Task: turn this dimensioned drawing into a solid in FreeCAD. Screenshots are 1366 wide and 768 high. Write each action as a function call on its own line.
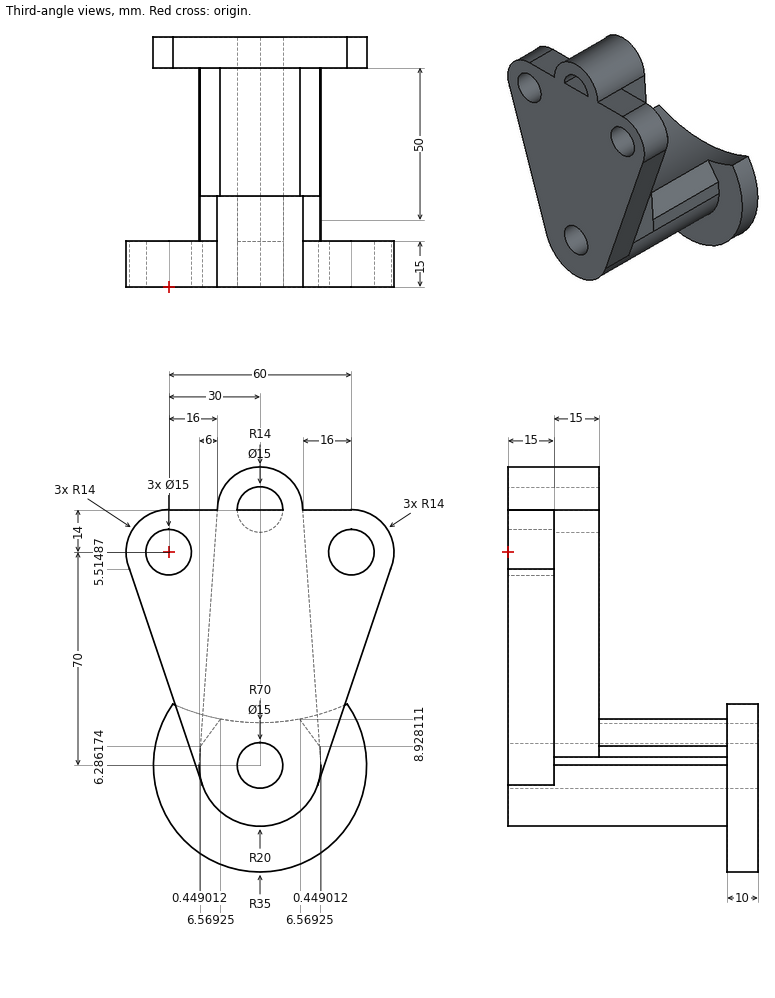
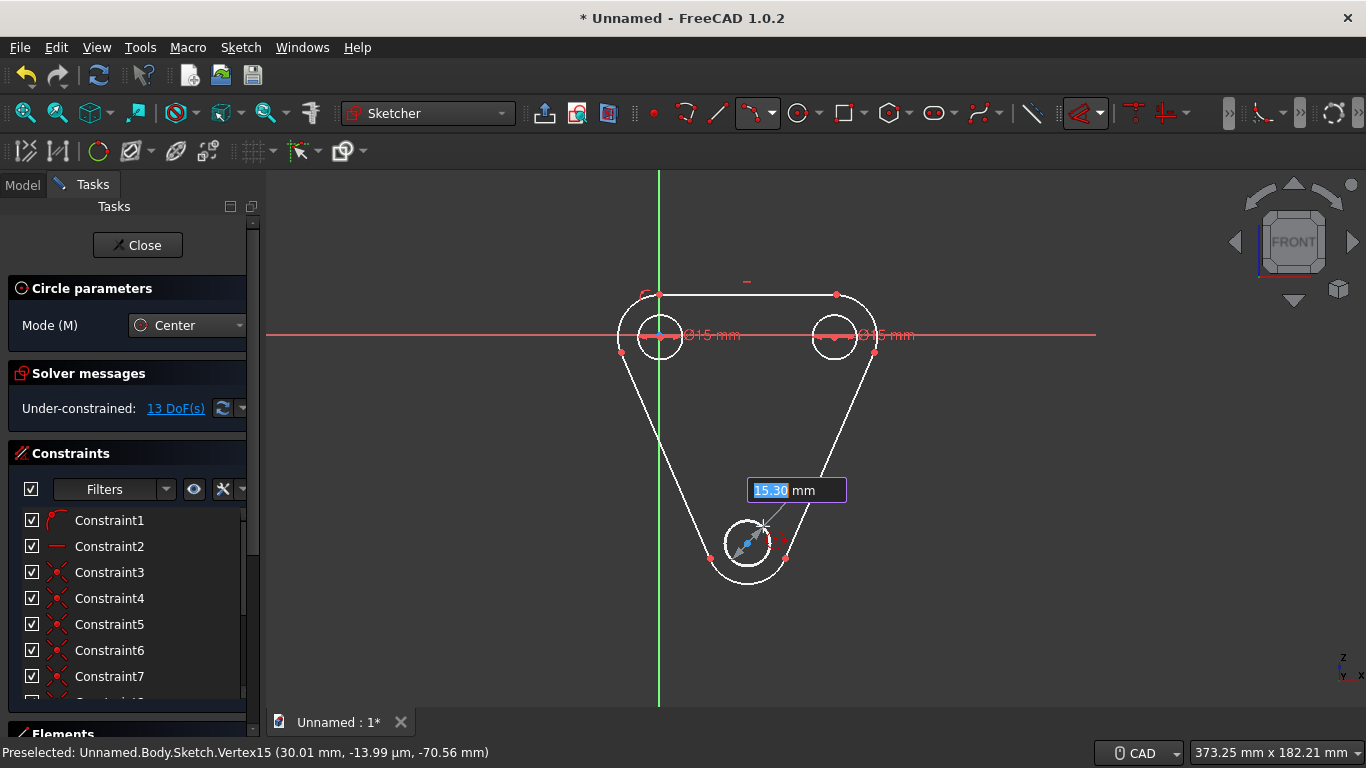
text(15)
key(Return)
key(Escape)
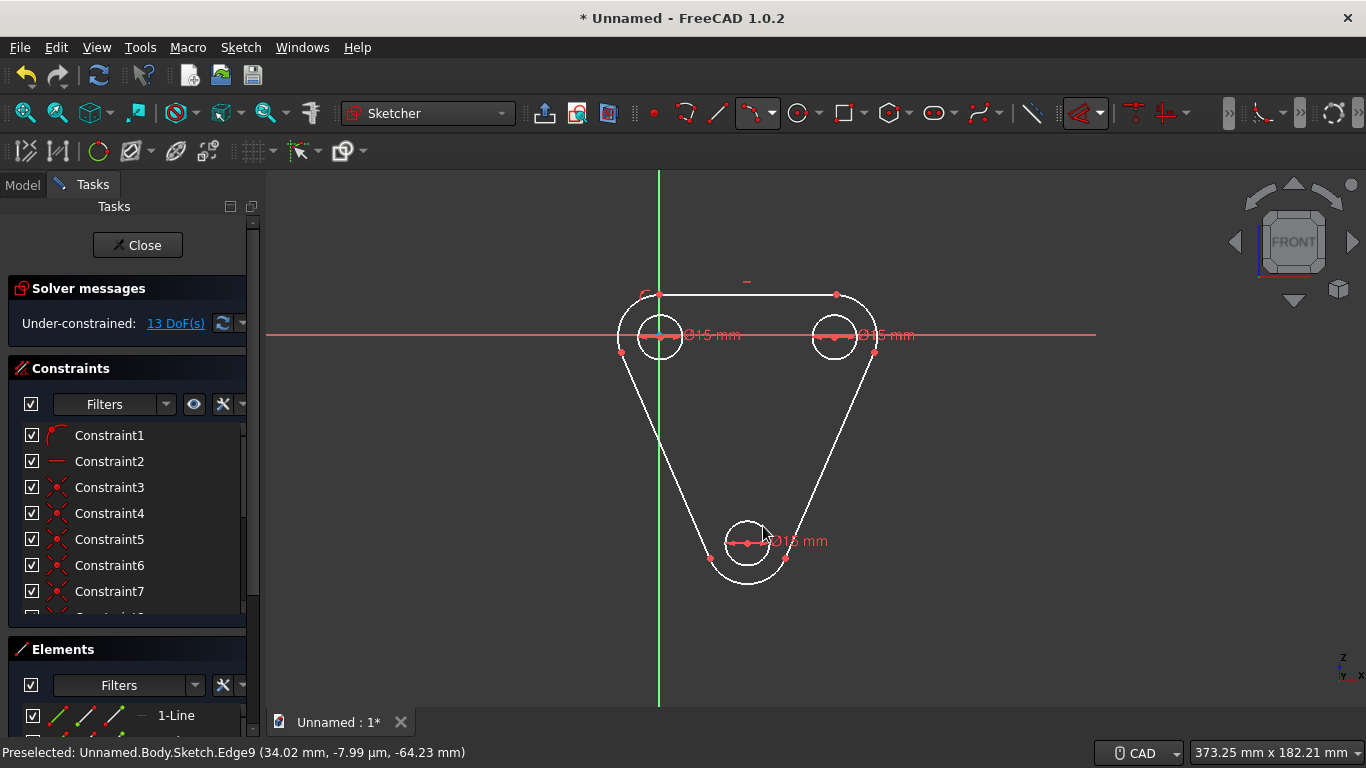
click(683, 497)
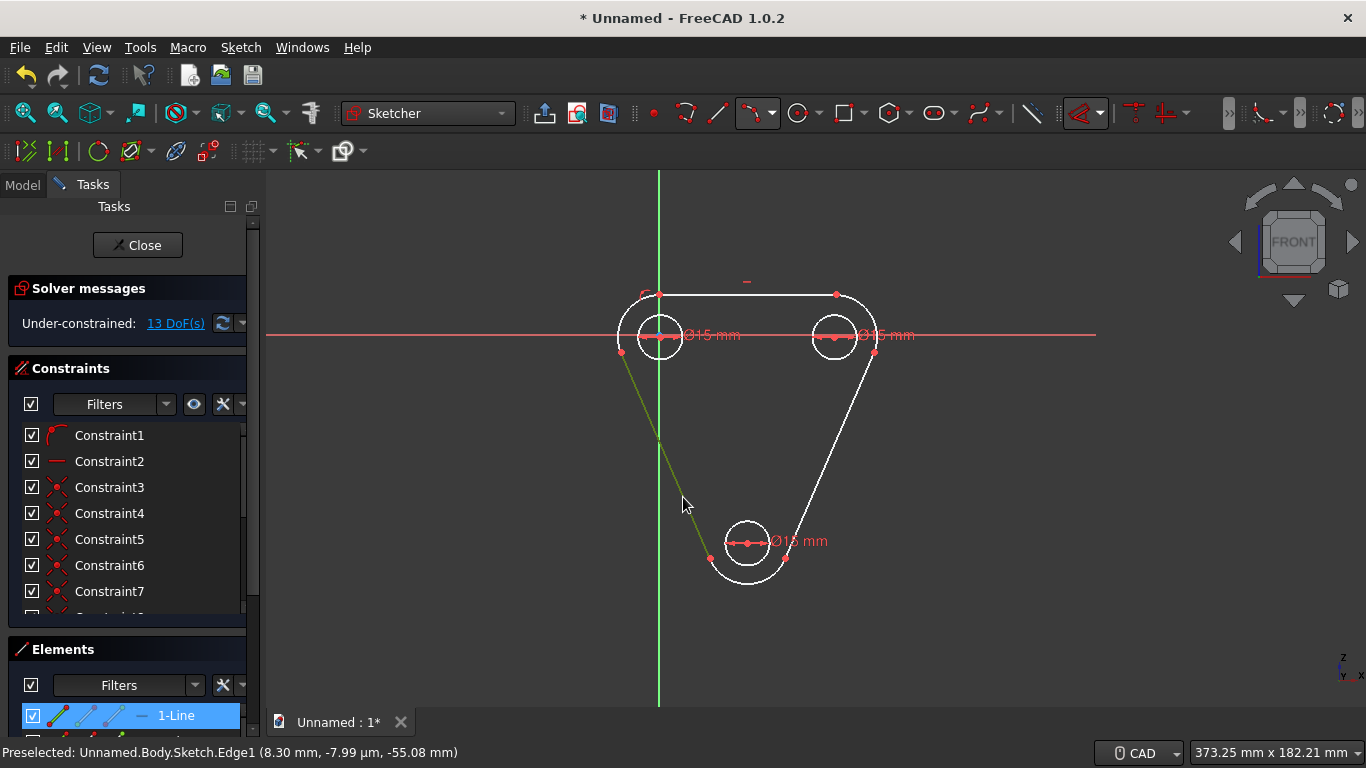
click(636, 303)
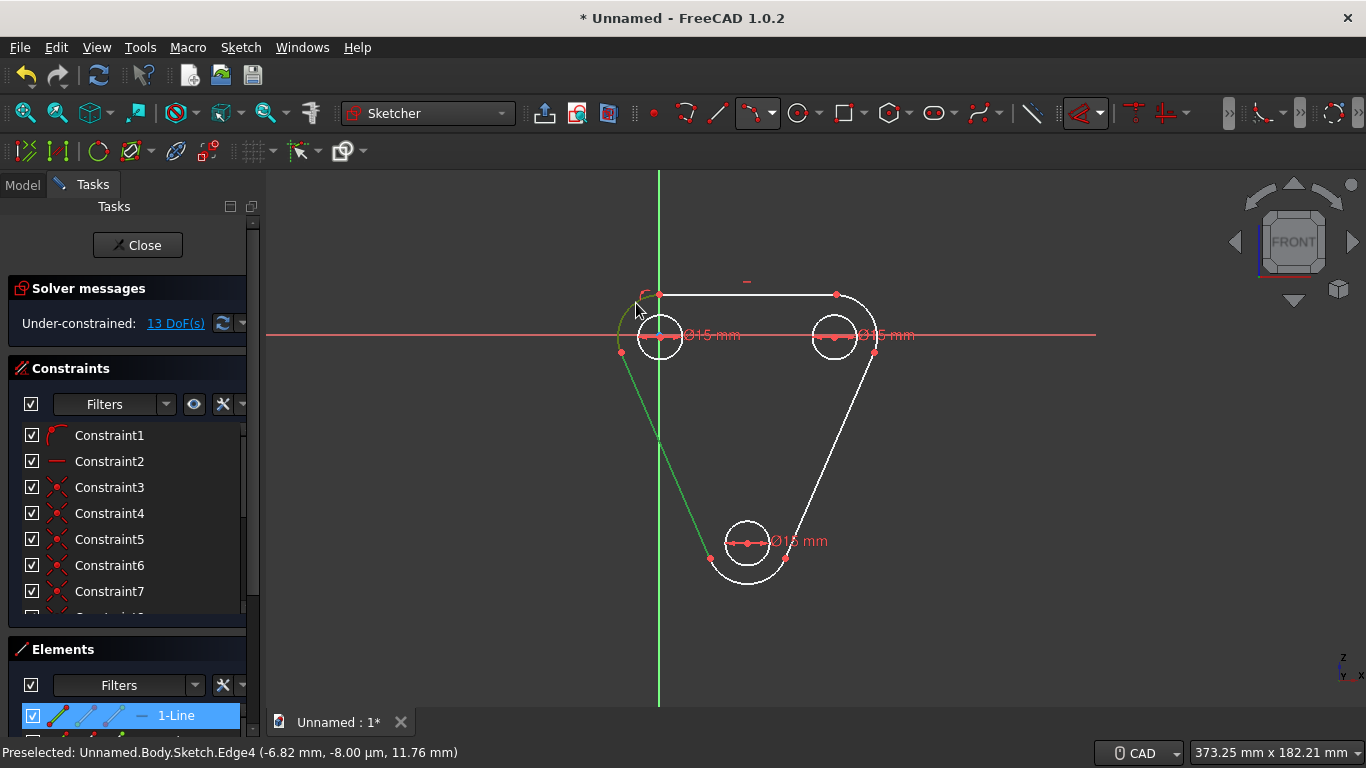
key(t)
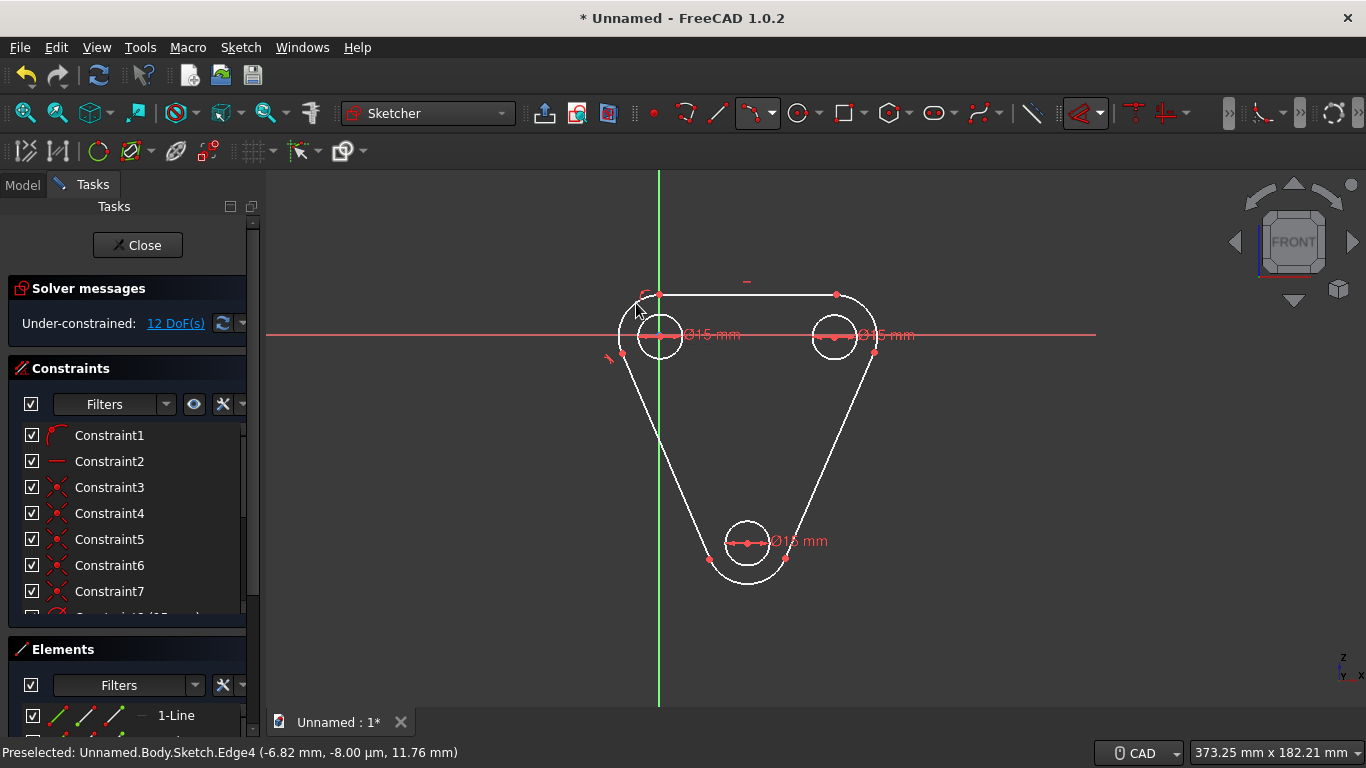
click(684, 497)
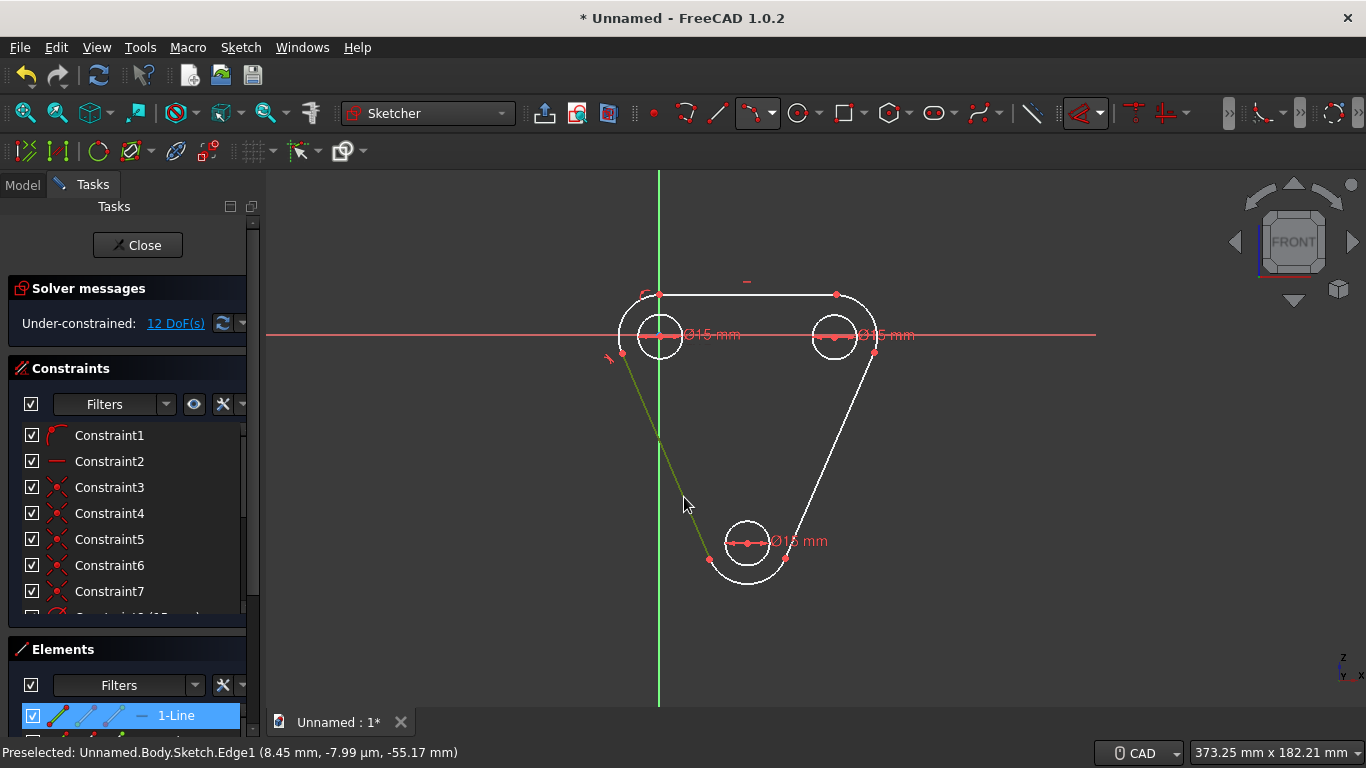
click(729, 580)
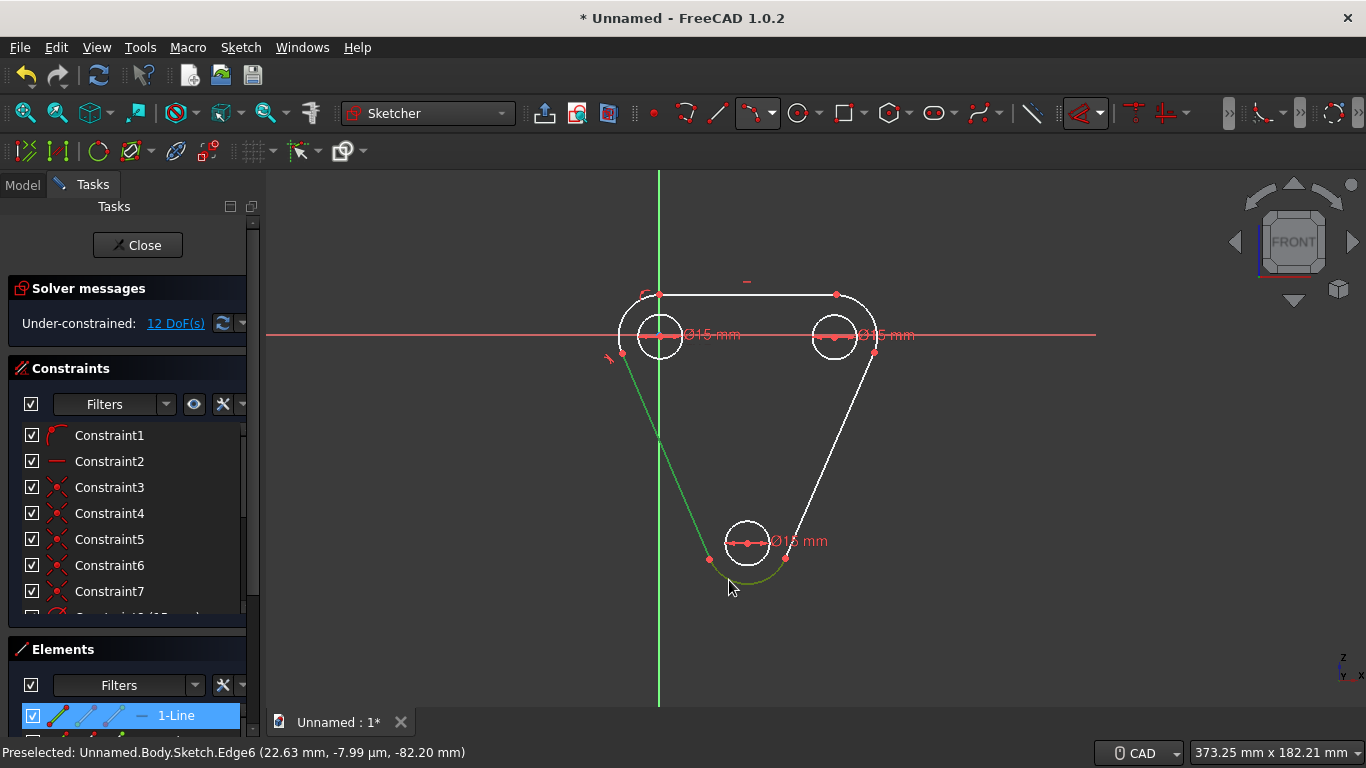
key(t)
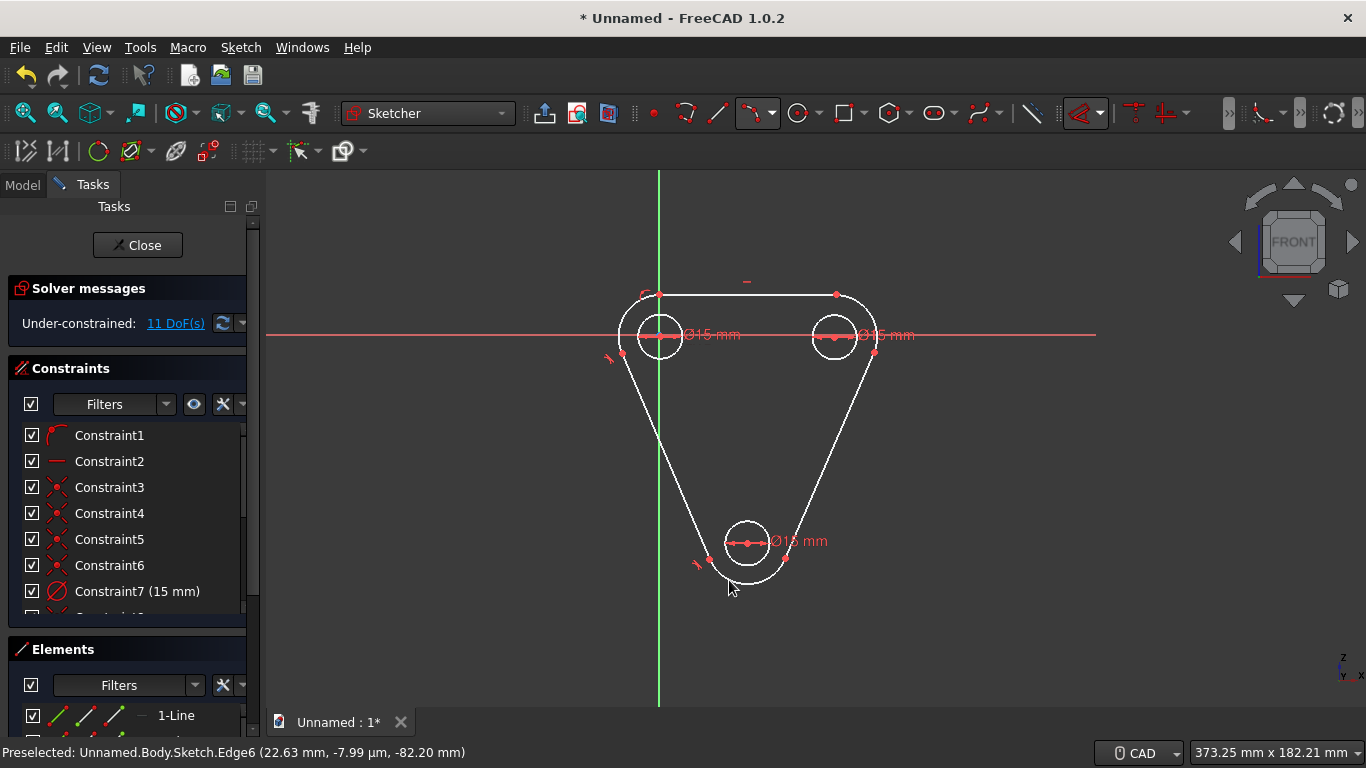
click(712, 295)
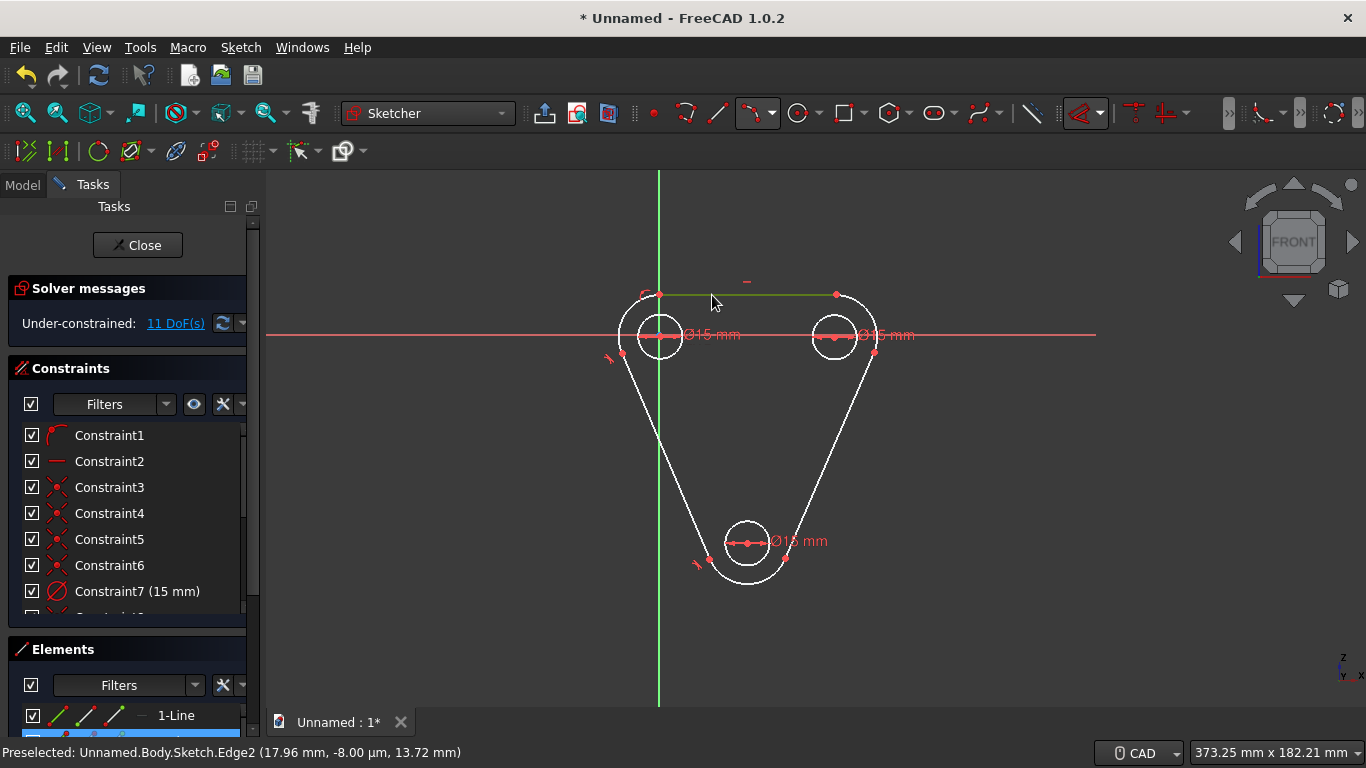
click(636, 303)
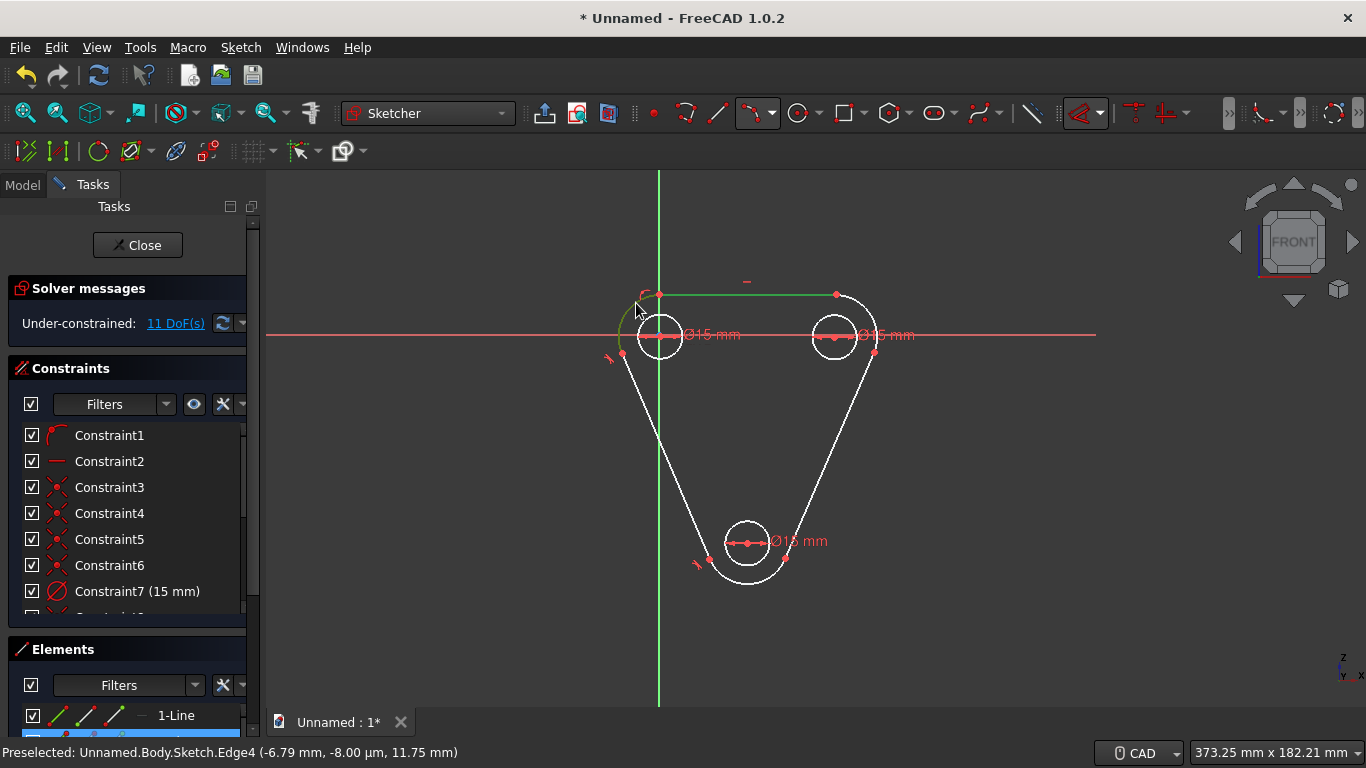
key(t)